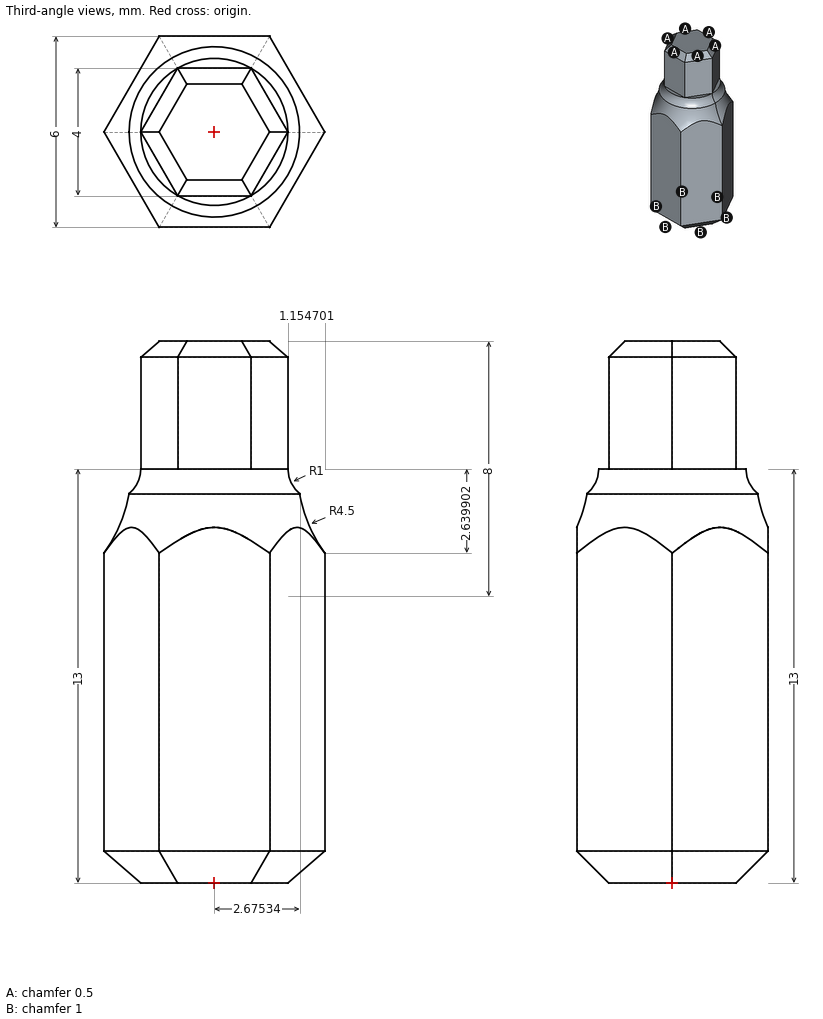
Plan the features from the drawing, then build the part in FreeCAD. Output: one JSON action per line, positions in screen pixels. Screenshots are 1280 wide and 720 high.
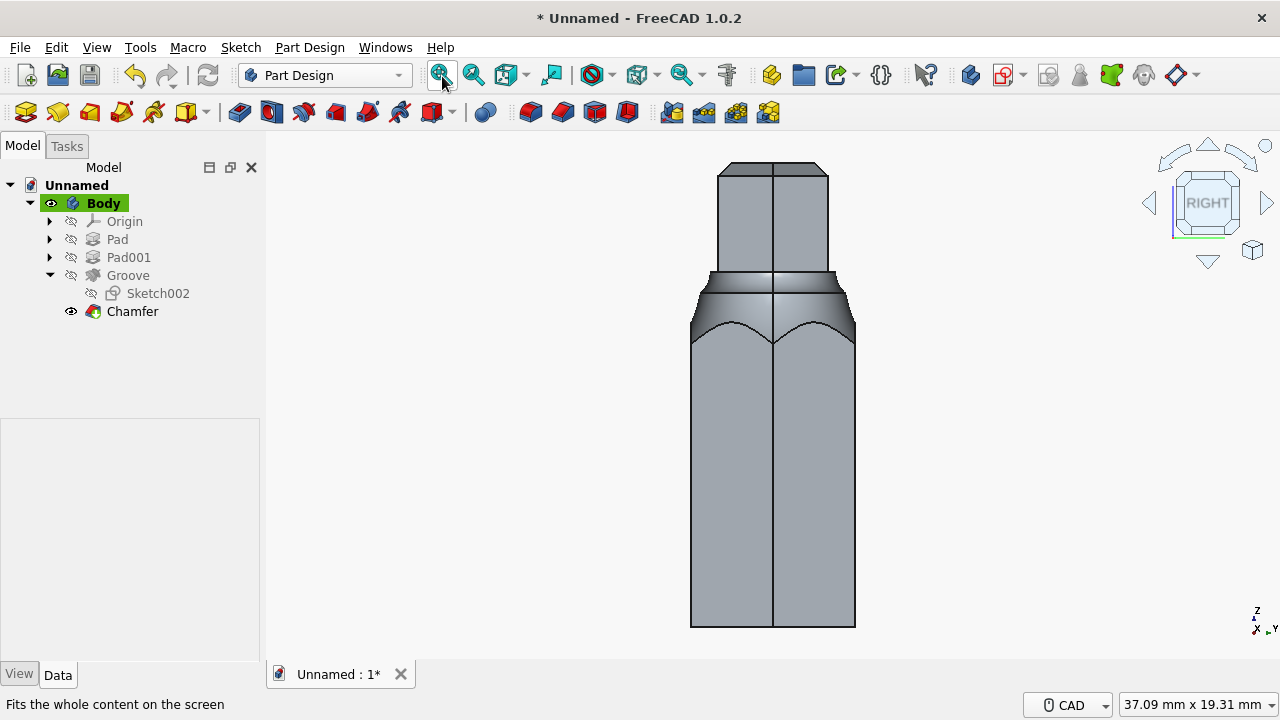
{"action": "key", "text": "5"}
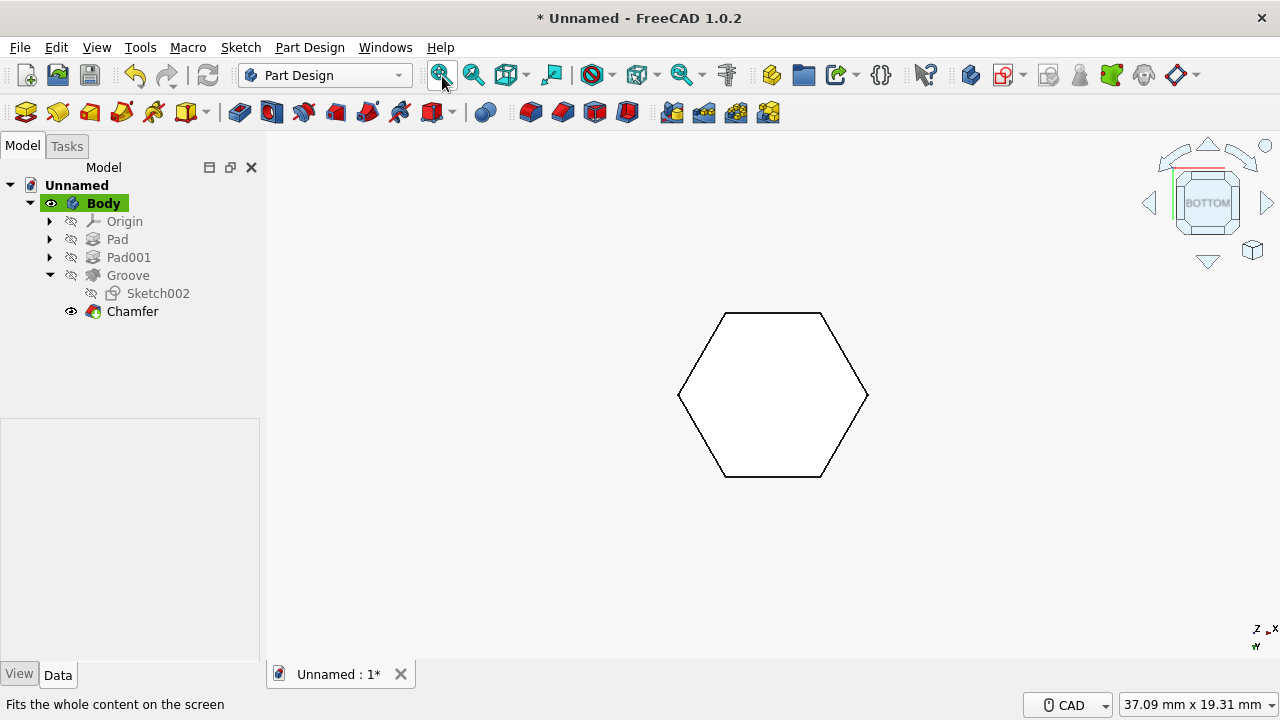
{"action": "left_click", "coordinate": [442, 76]}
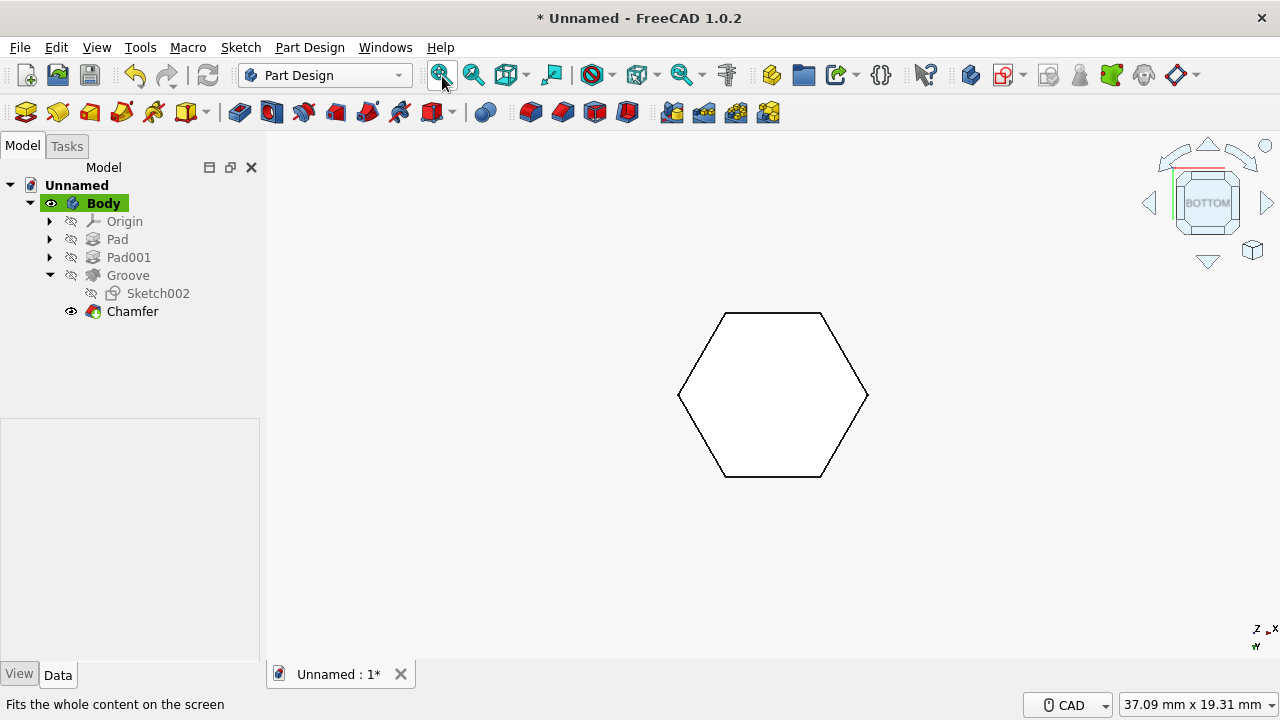
{"action": "left_click", "coordinate": [773, 394]}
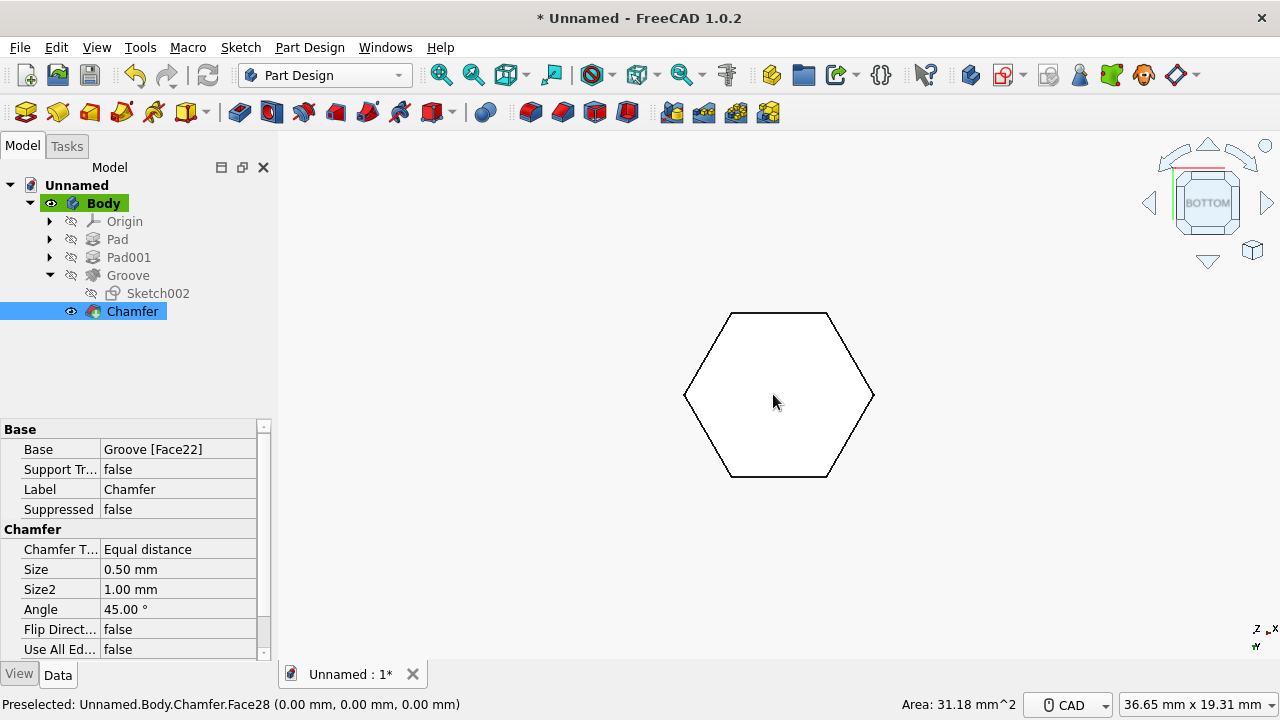
{"action": "left_click", "coordinate": [564, 112]}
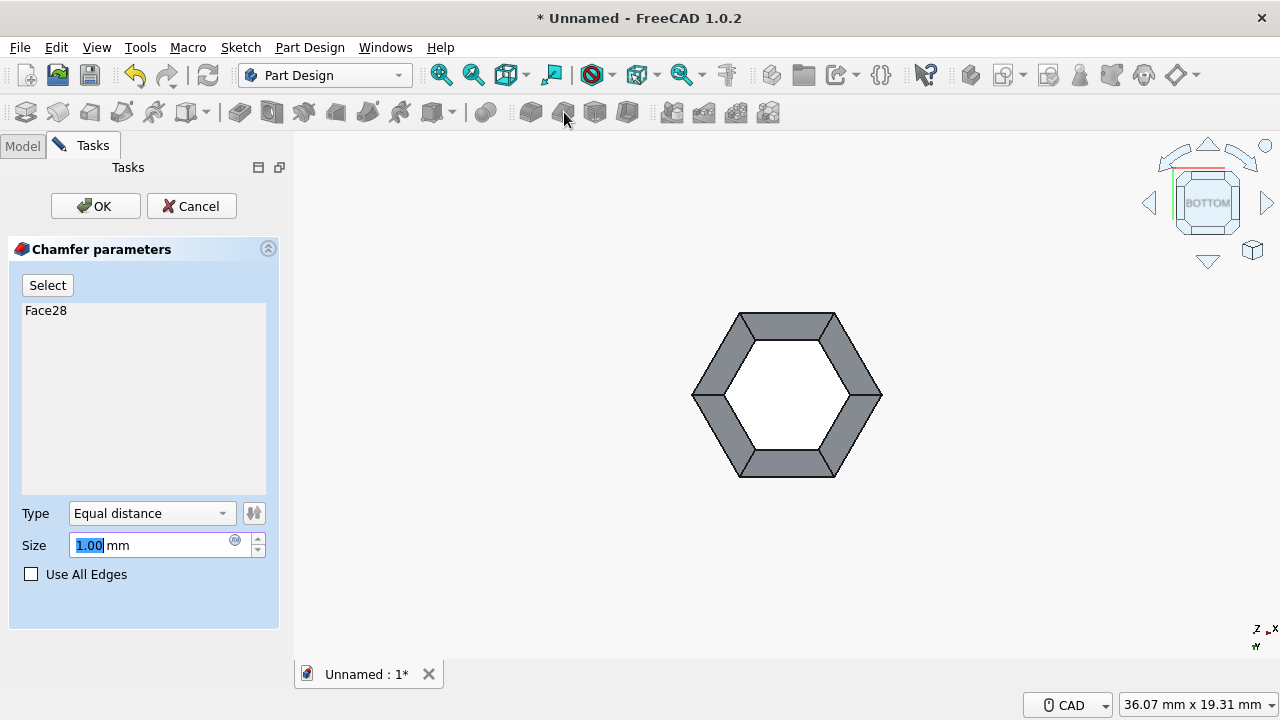
{"action": "type", "text": "1"}
{"action": "key", "text": "Tab"}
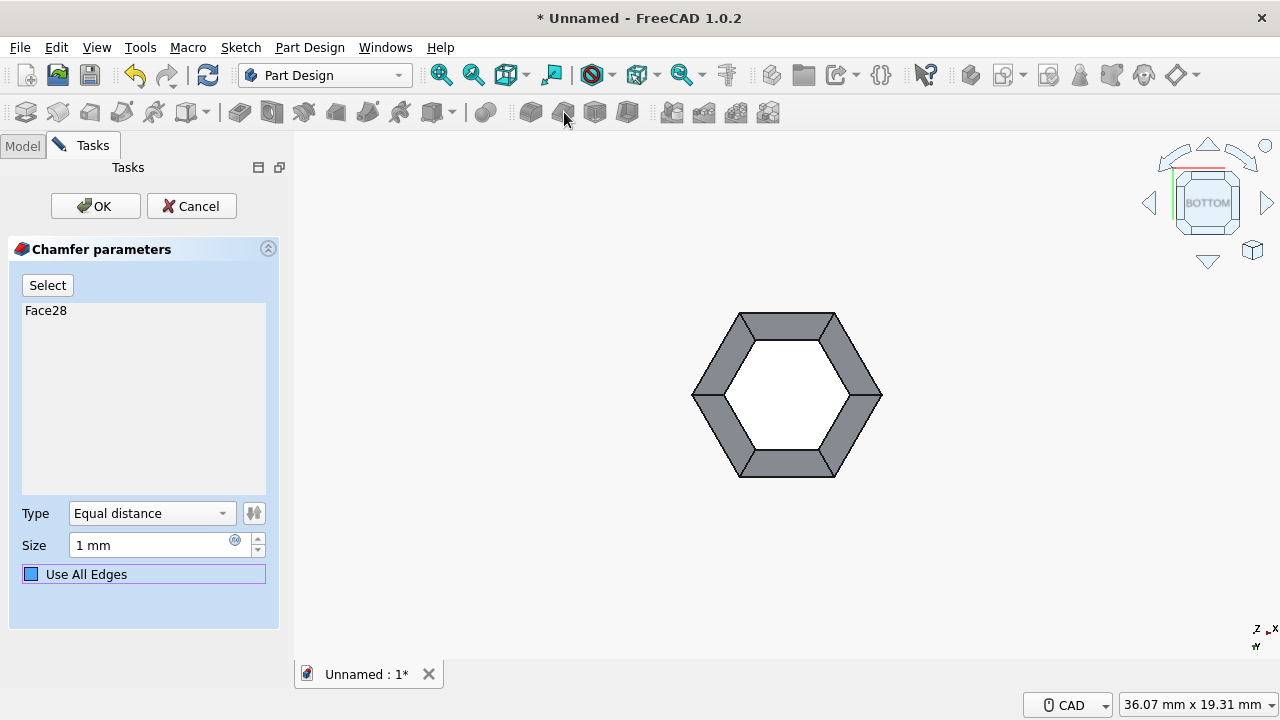
{"action": "left_click", "coordinate": [96, 206]}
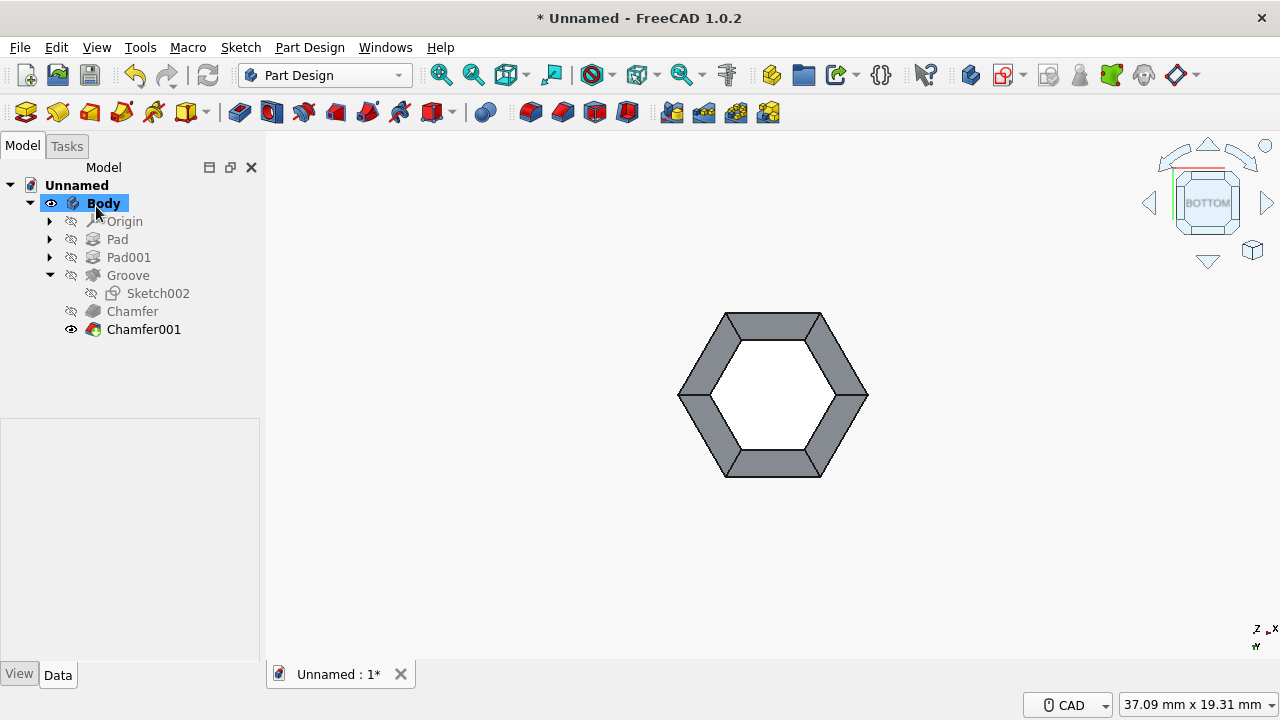
{"action": "key", "text": "0"}